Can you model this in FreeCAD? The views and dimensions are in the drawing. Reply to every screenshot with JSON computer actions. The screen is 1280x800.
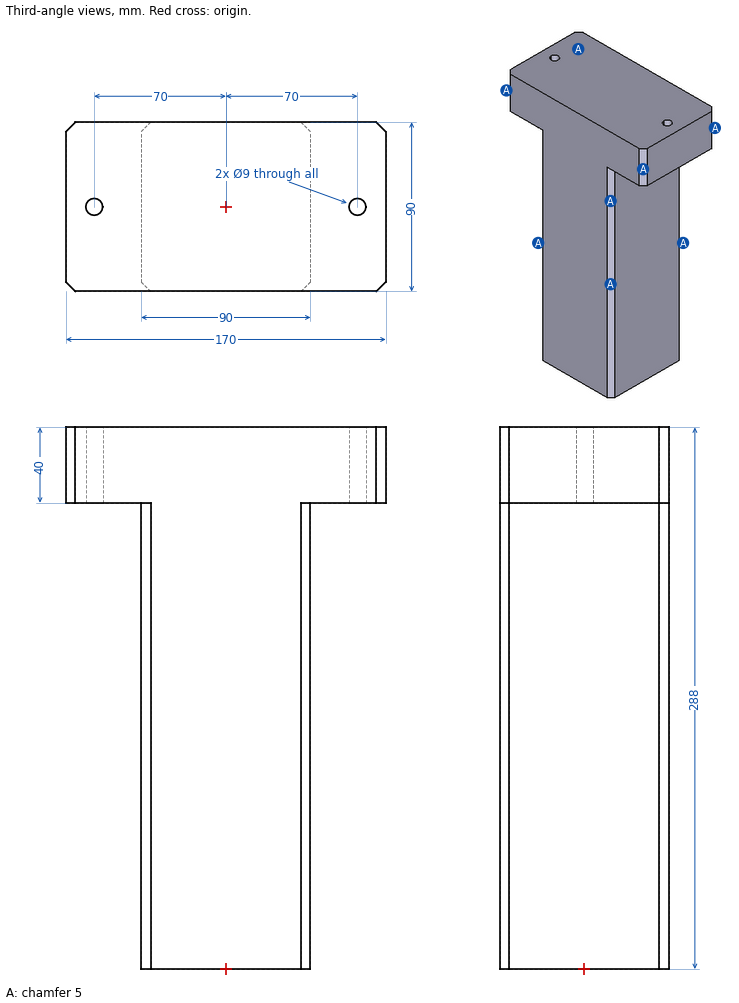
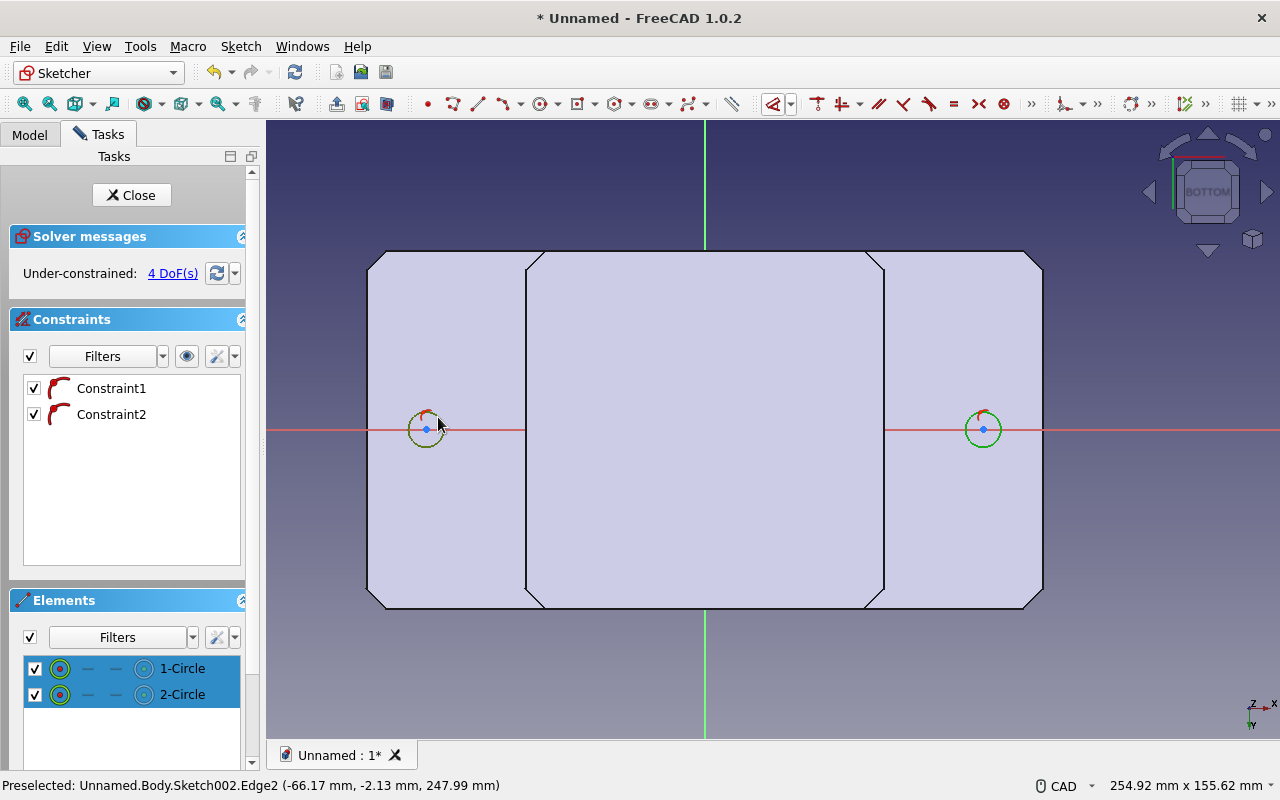
{"action": "left_click", "coordinate": [954, 104]}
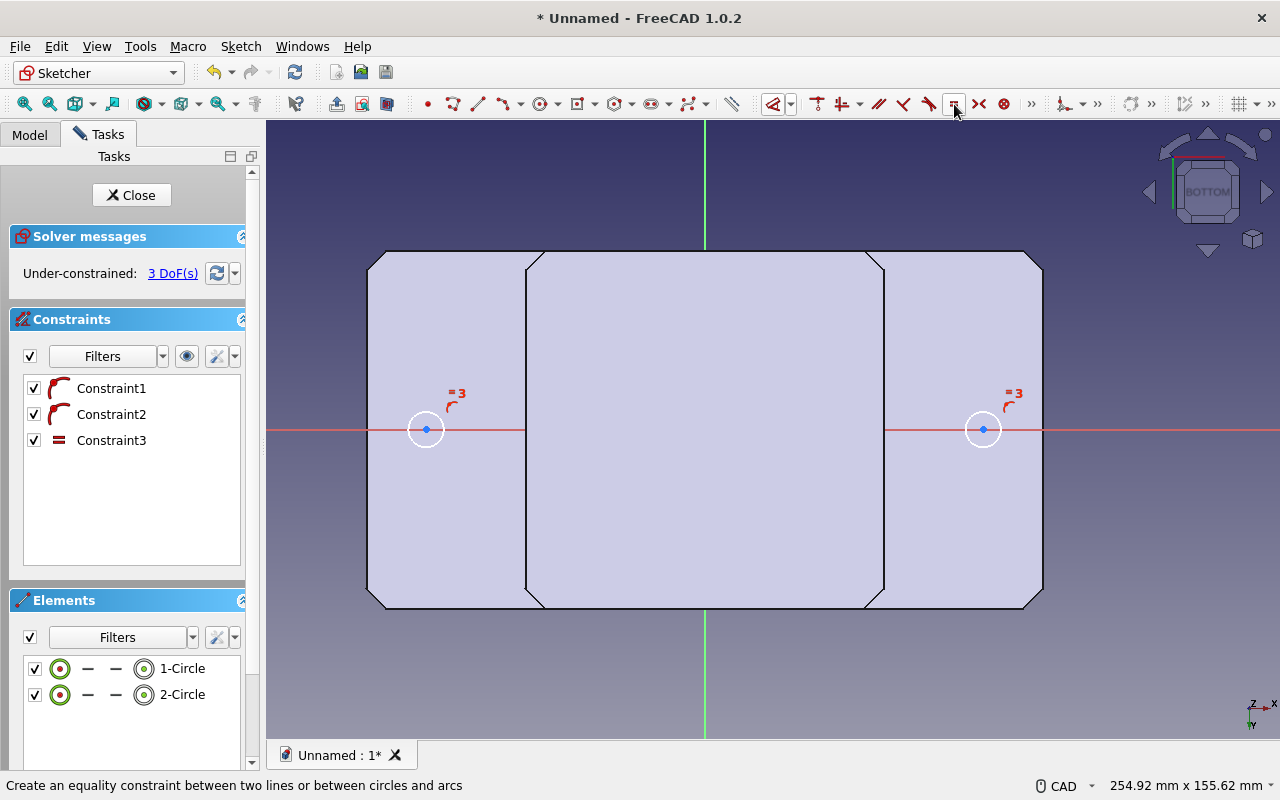
{"action": "left_click", "coordinate": [996, 417]}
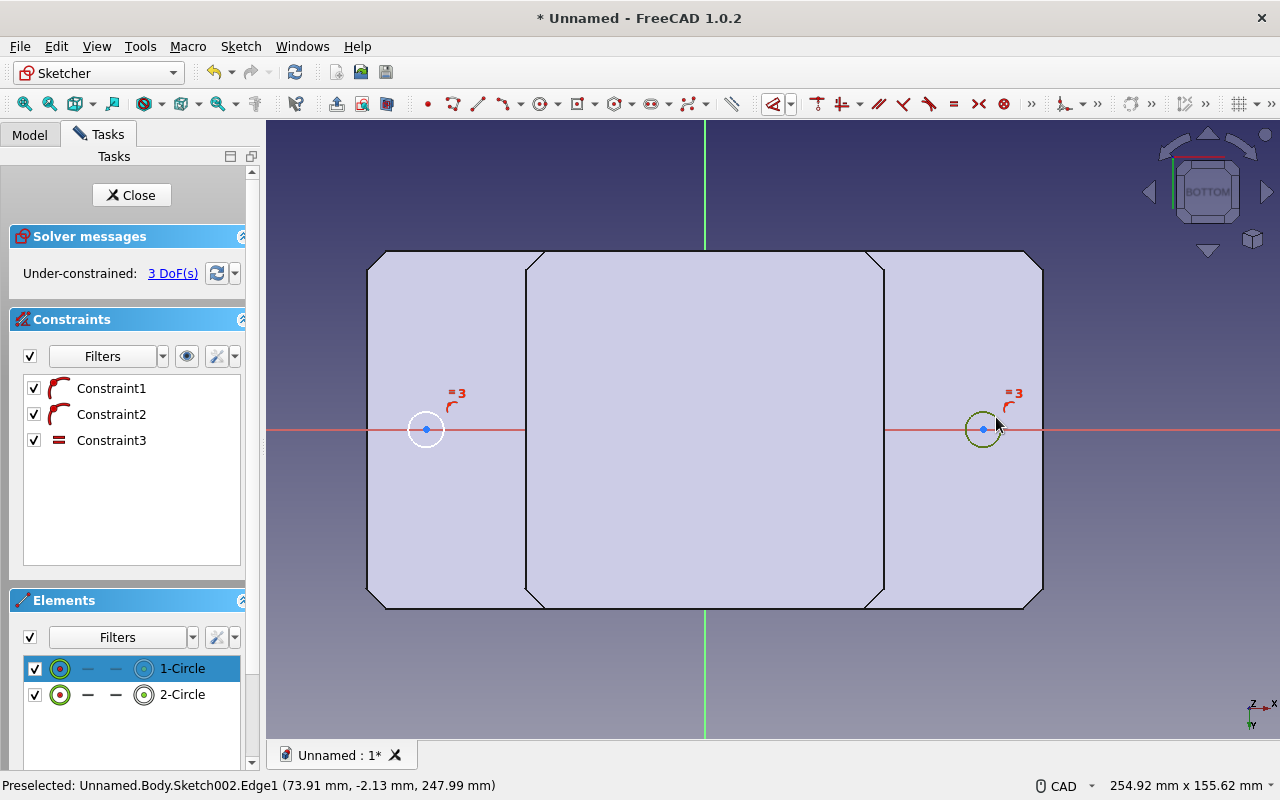
{"action": "key", "text": "k o"}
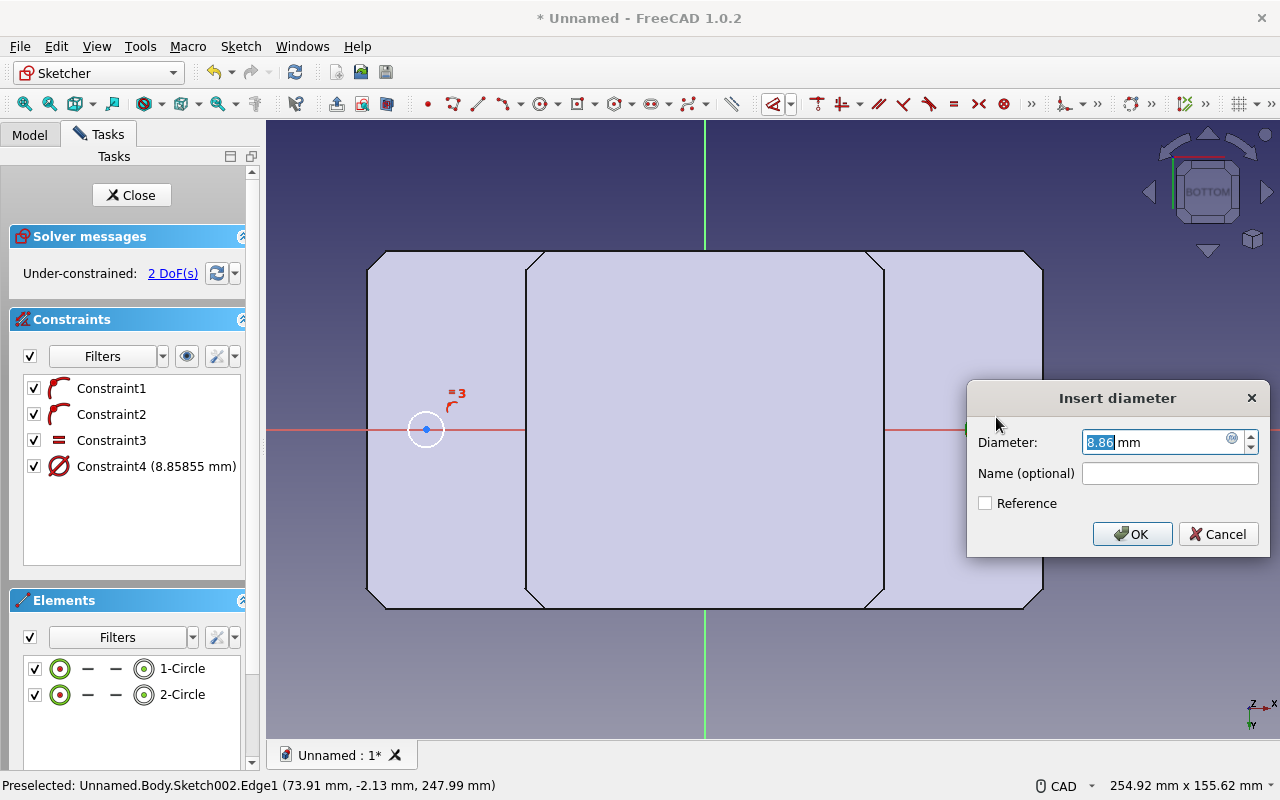
{"action": "type", "text": "9"}
{"action": "key", "text": "Return"}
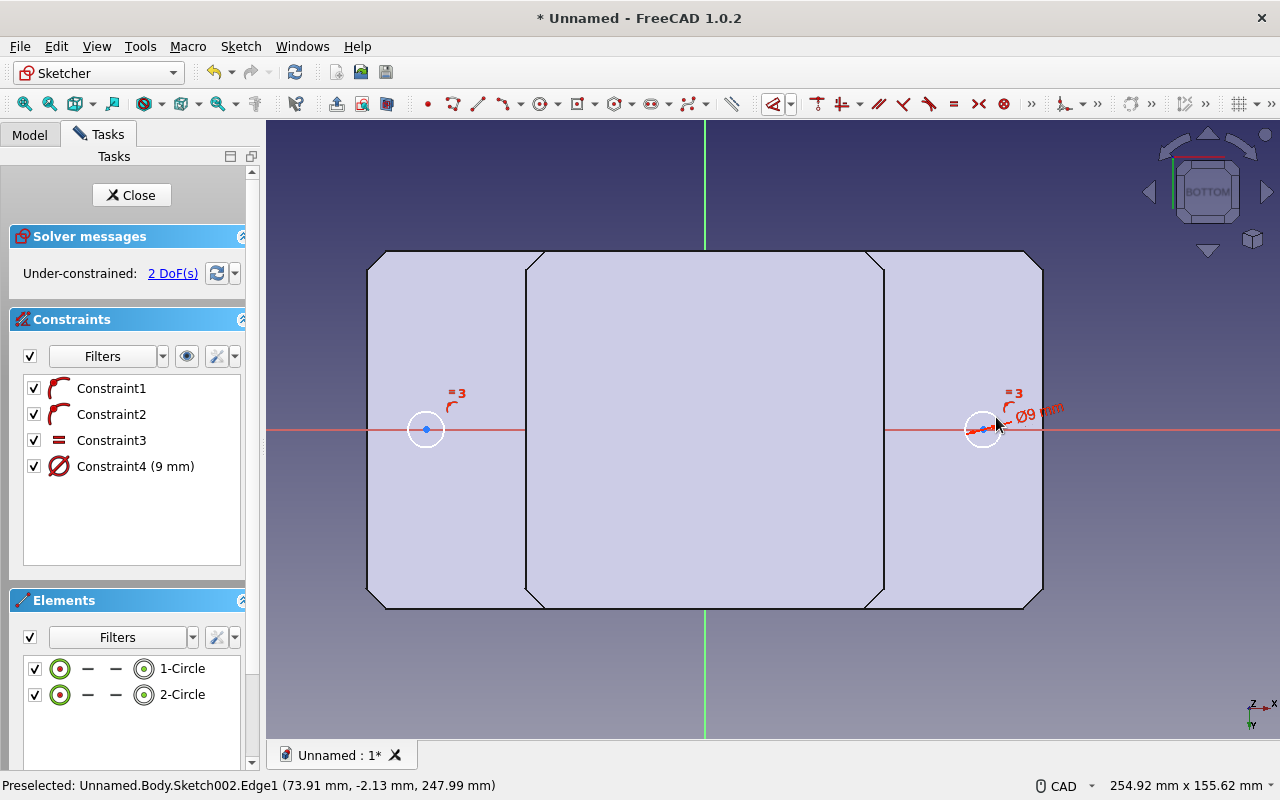
{"action": "left_click", "coordinate": [983, 430]}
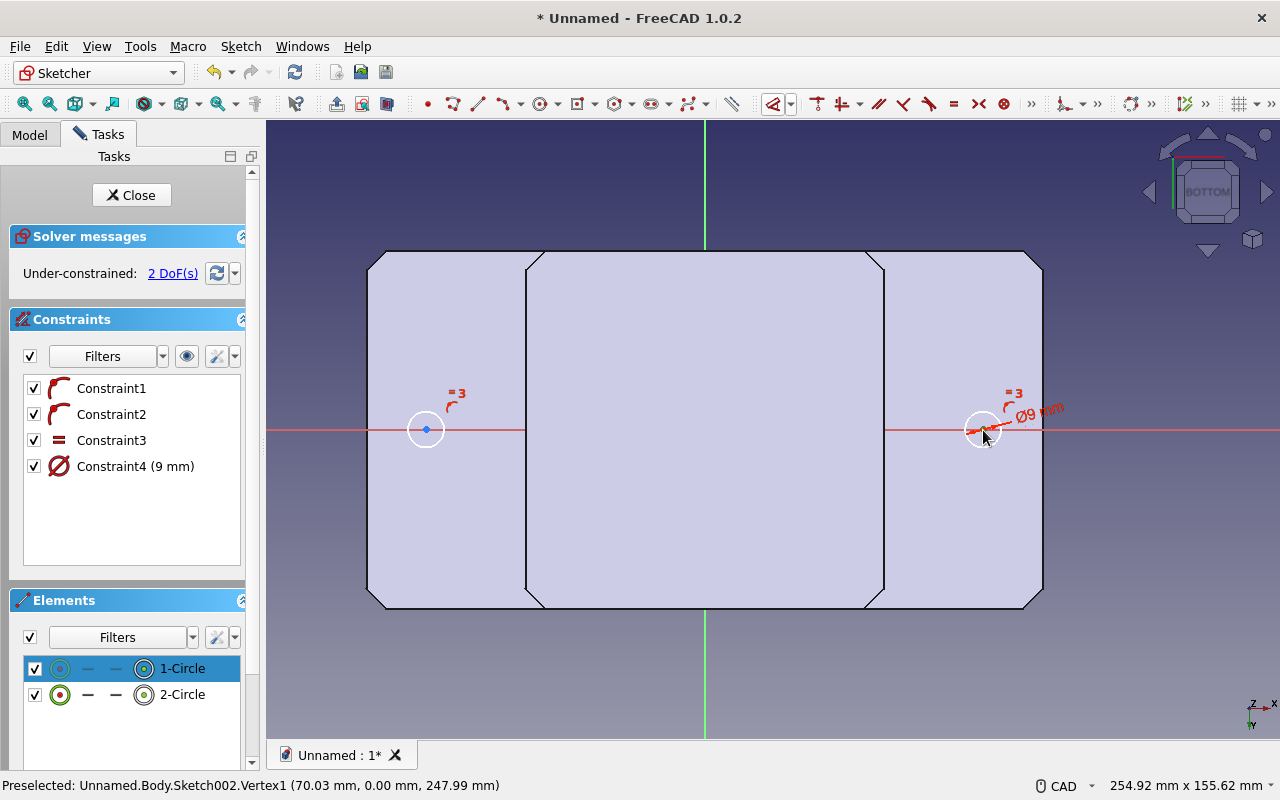
{"action": "left_click", "coordinate": [790, 104]}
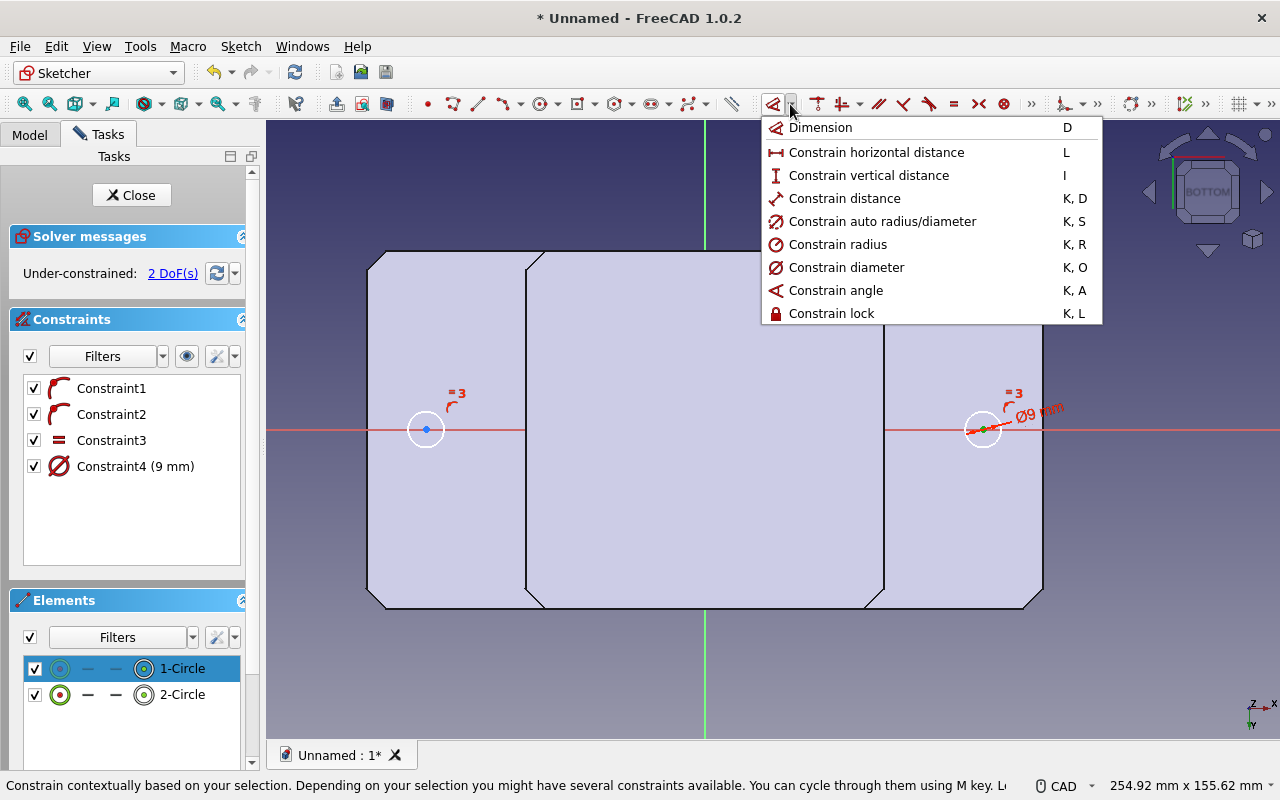
{"action": "left_click", "coordinate": [932, 152]}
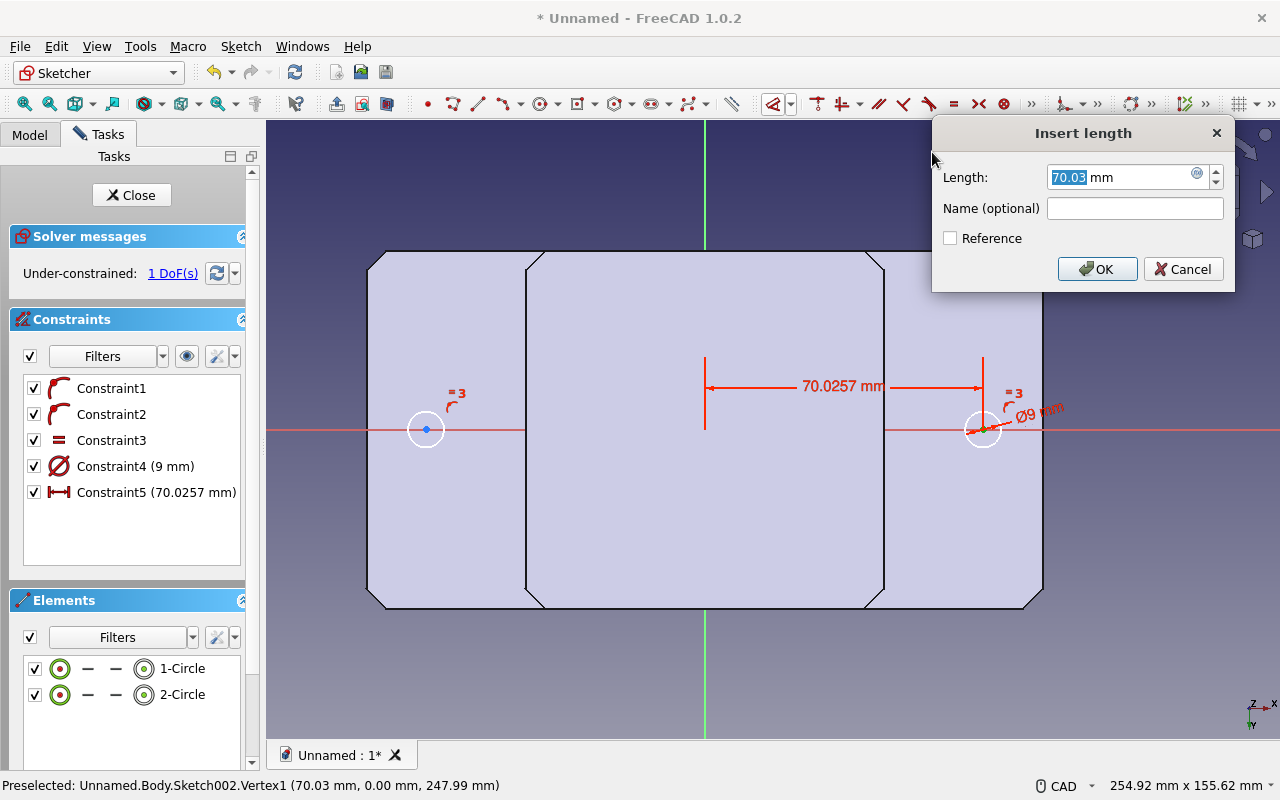
{"action": "type", "text": "70"}
{"action": "key", "text": "Return"}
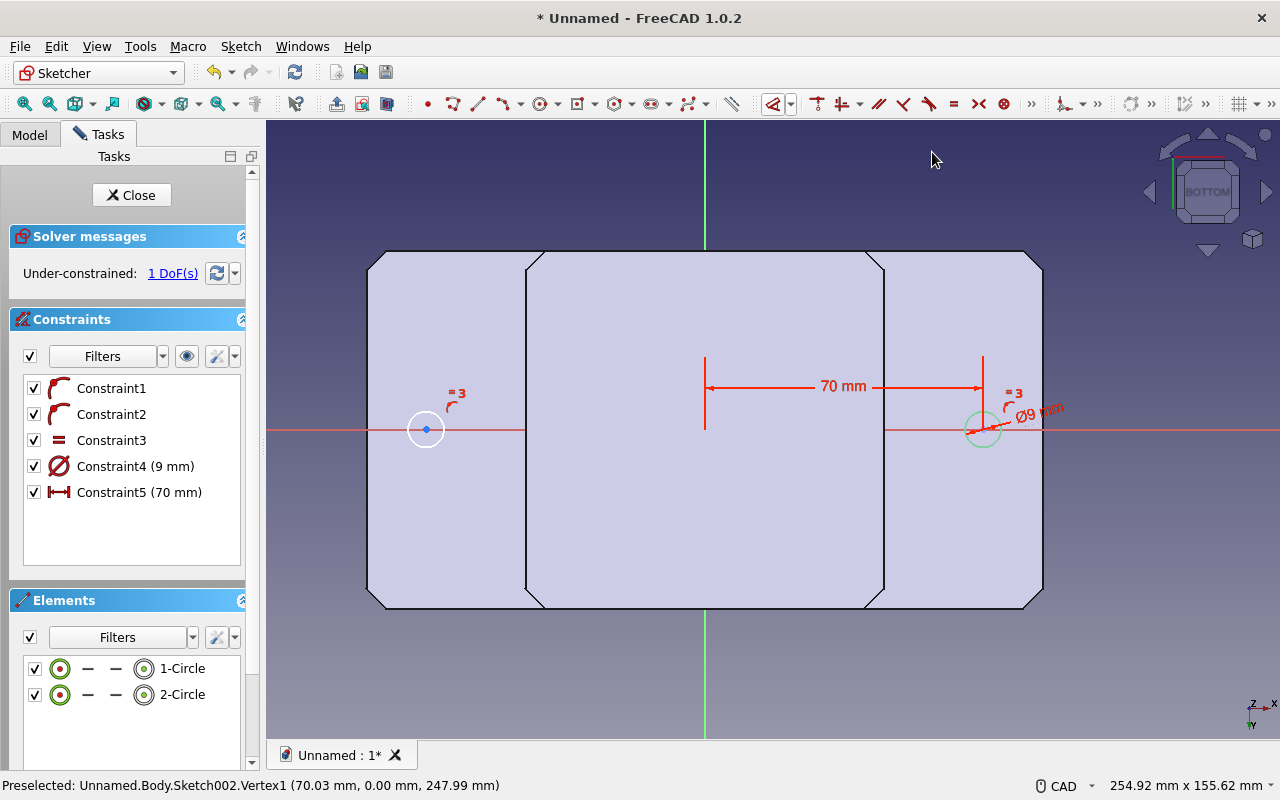
{"action": "left_click", "coordinate": [426, 430]}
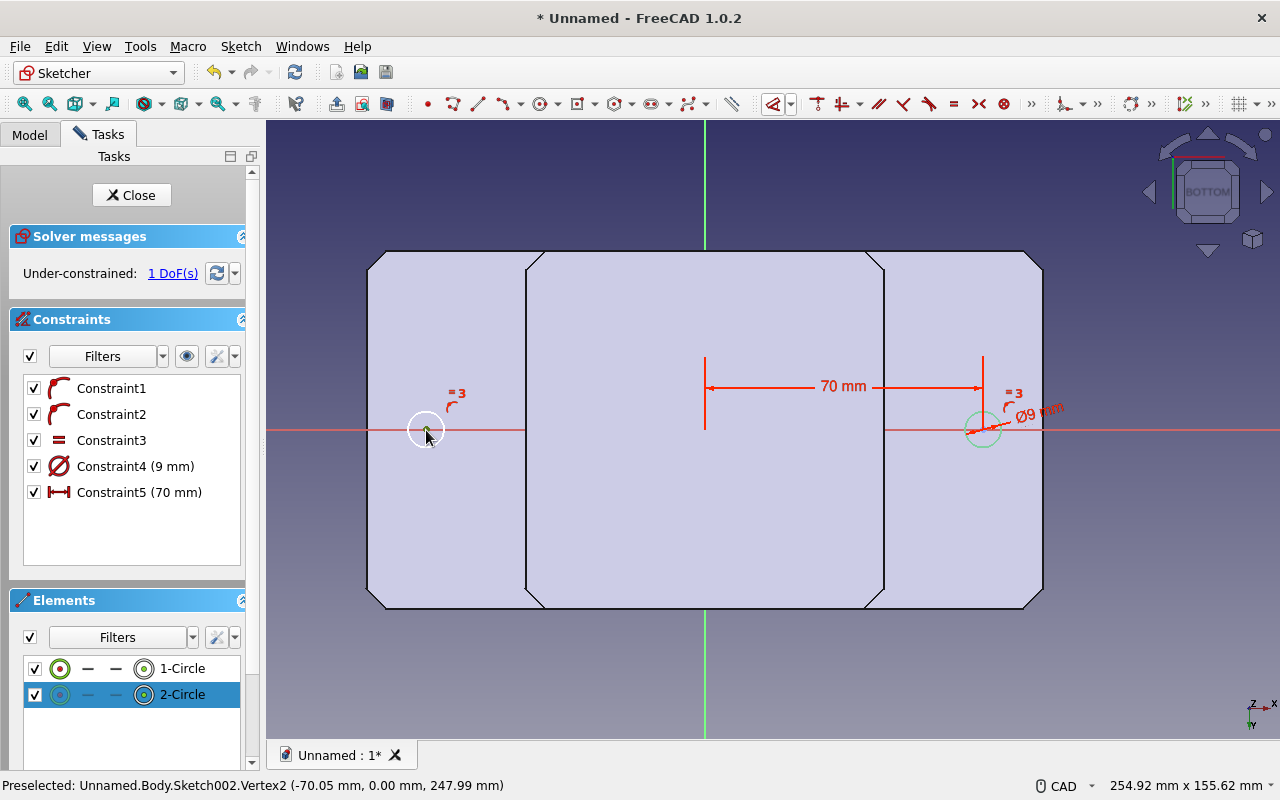
{"action": "left_click", "coordinate": [790, 104]}